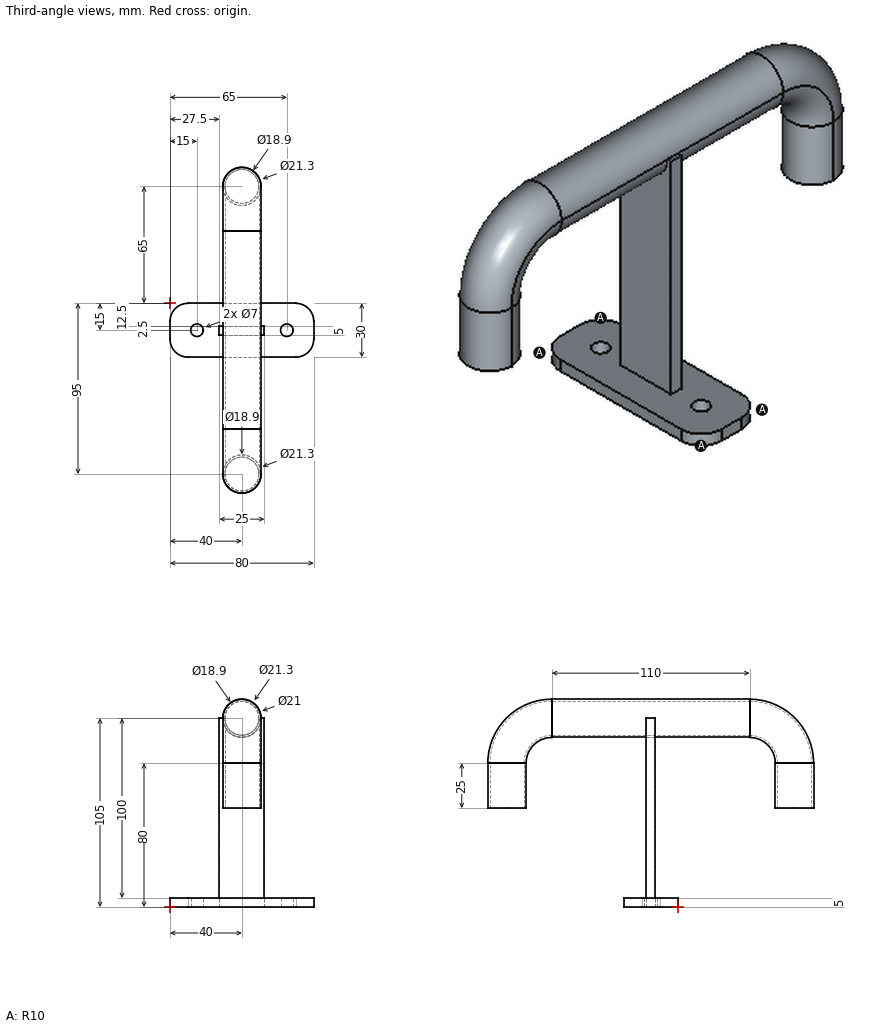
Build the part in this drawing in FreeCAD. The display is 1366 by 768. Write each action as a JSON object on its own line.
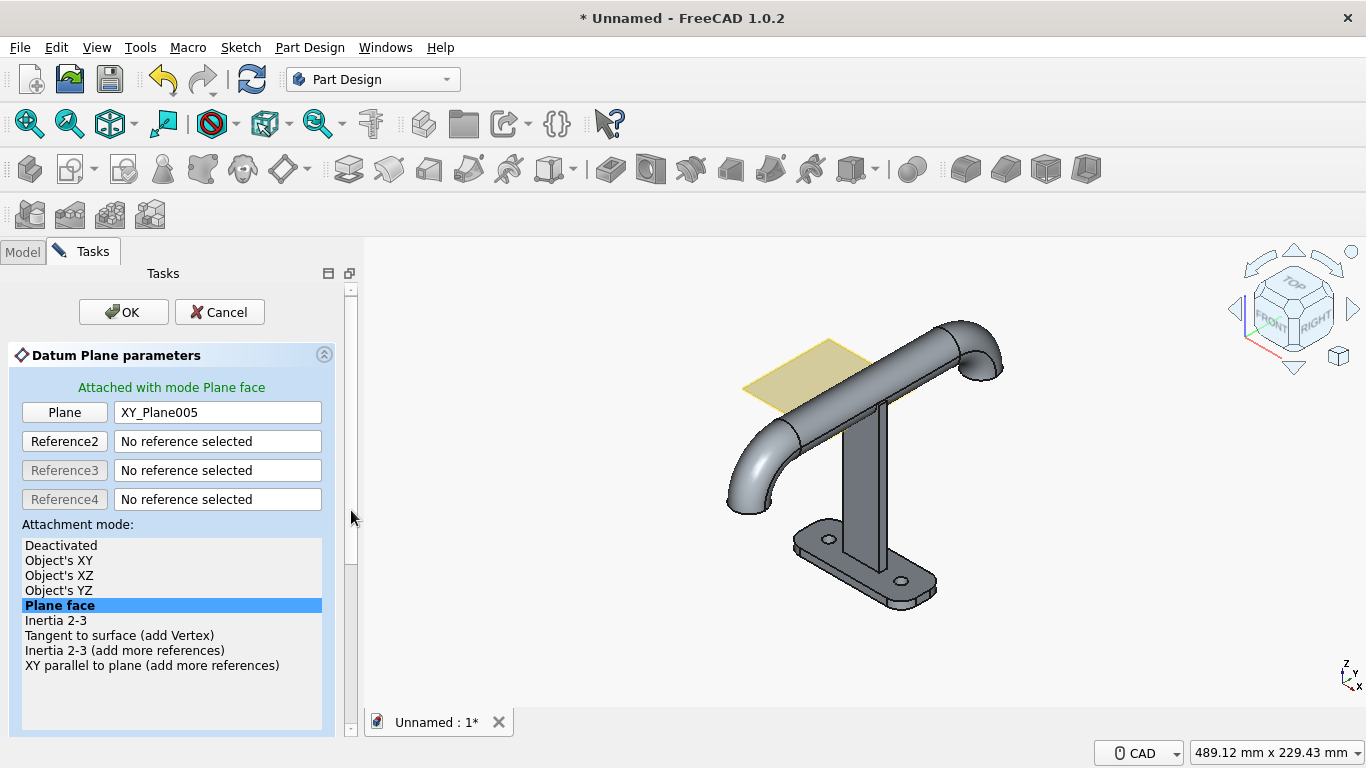
{"action": "left_click", "coordinate": [124, 312]}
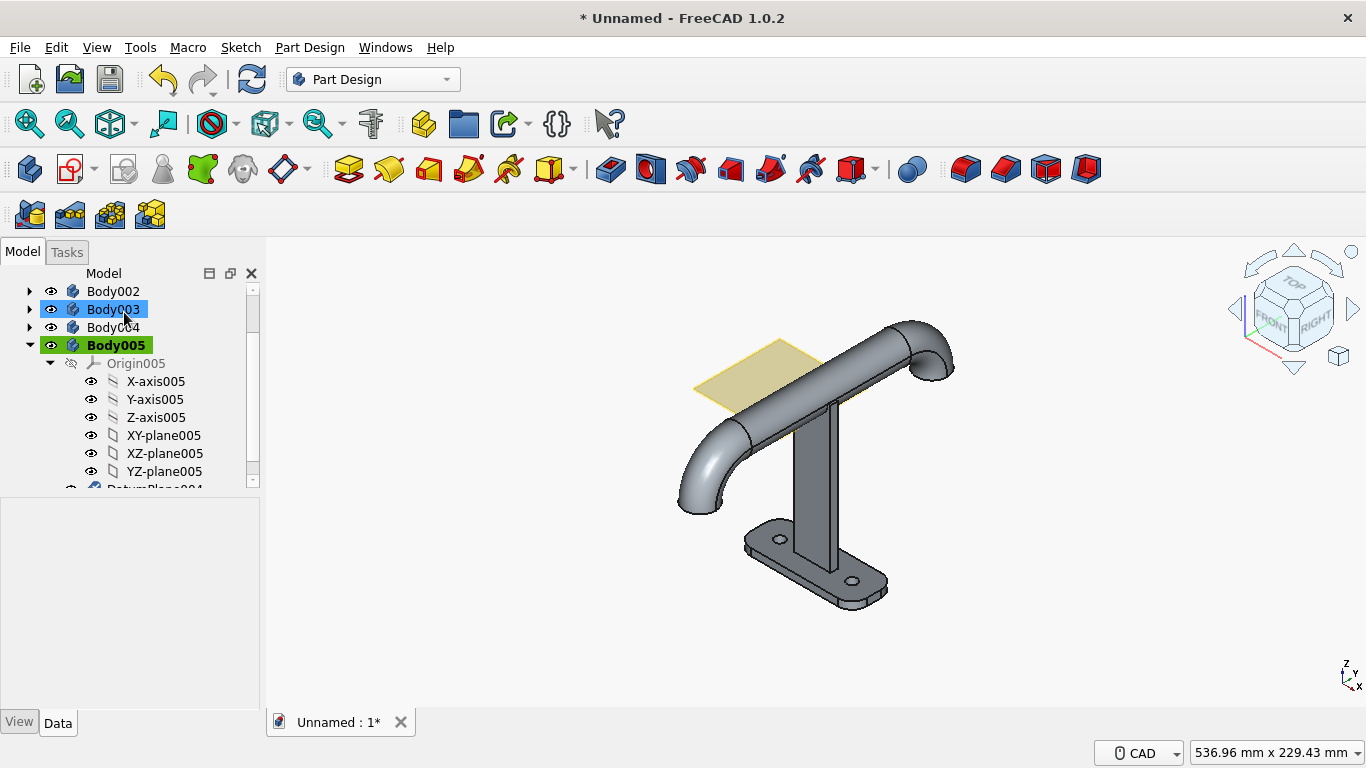
{"action": "scroll", "coordinate": [120, 377], "scroll_direction": "down", "scroll_amount": 3}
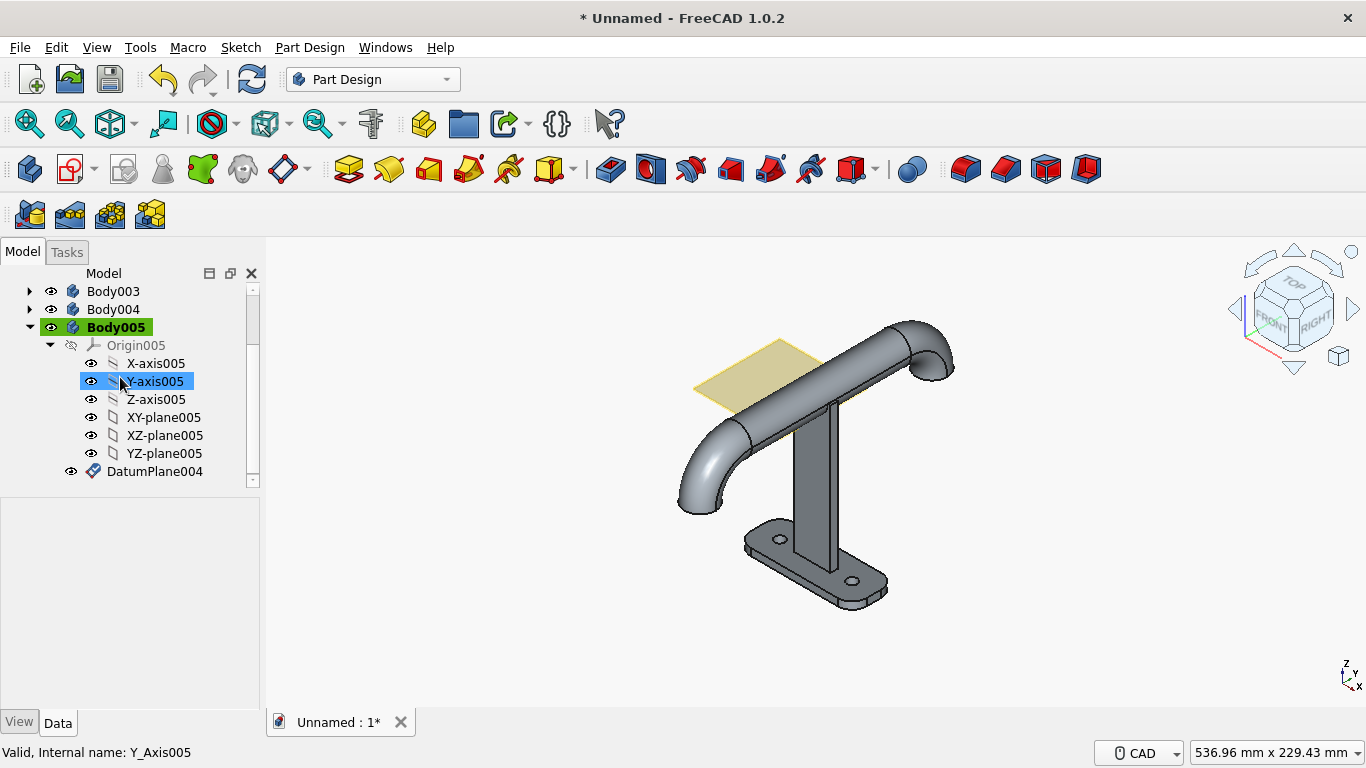
{"action": "left_click", "coordinate": [116, 471]}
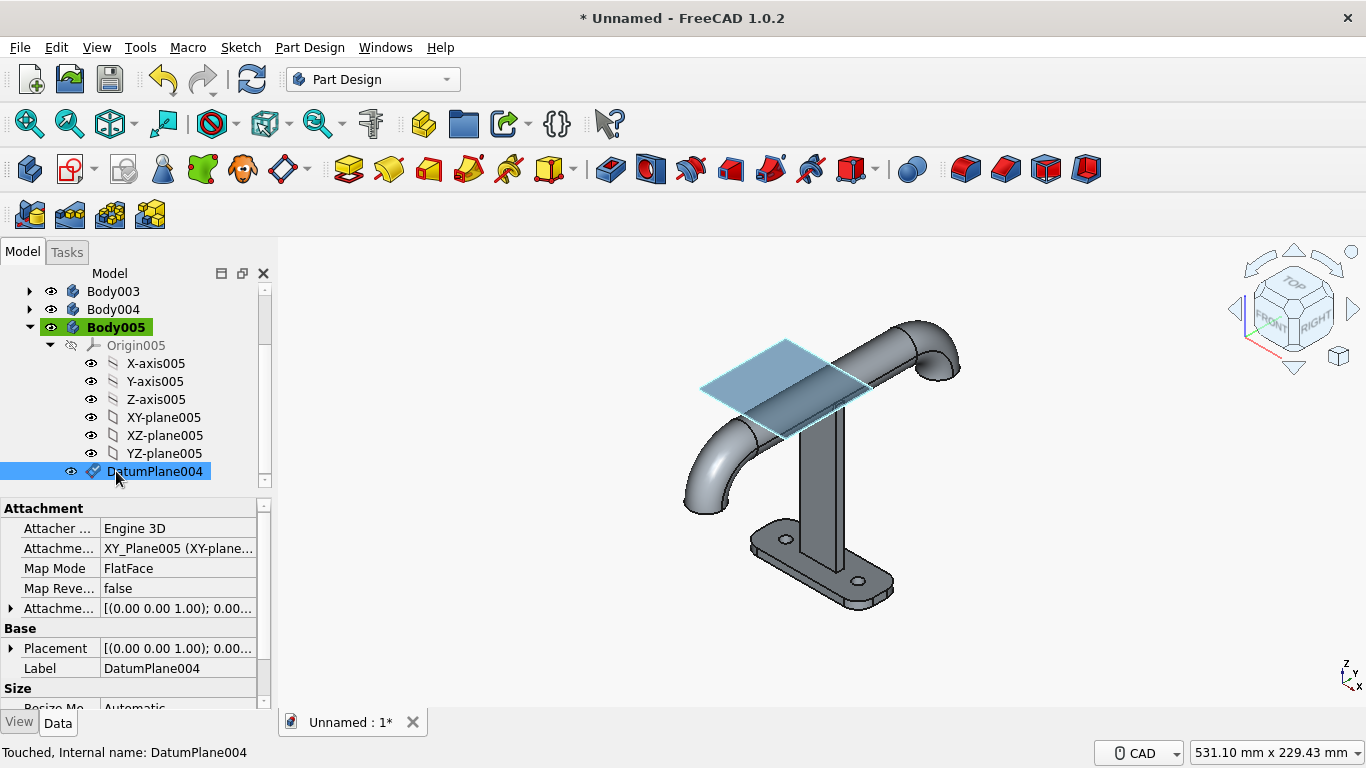
{"action": "left_click", "coordinate": [70, 170]}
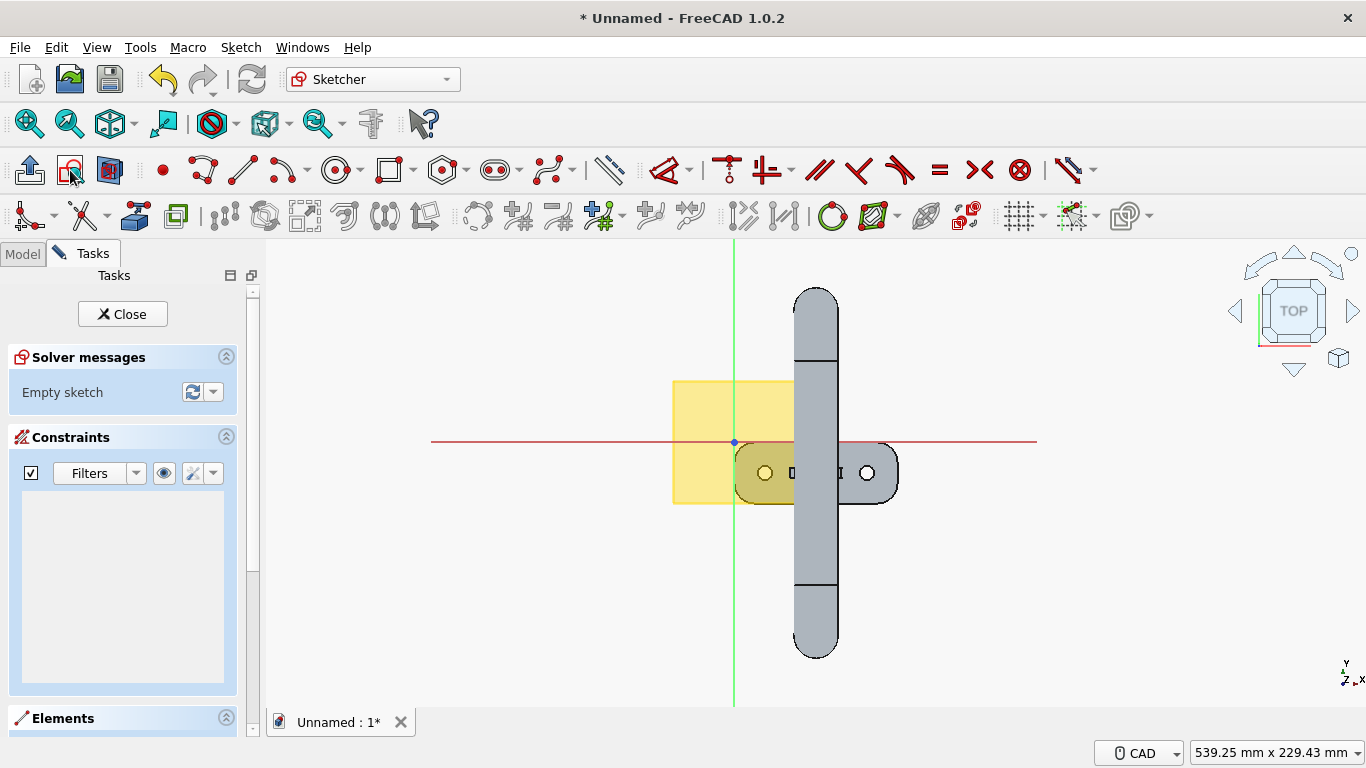
{"action": "scroll", "coordinate": [827, 662], "scroll_direction": "up", "scroll_amount": 10}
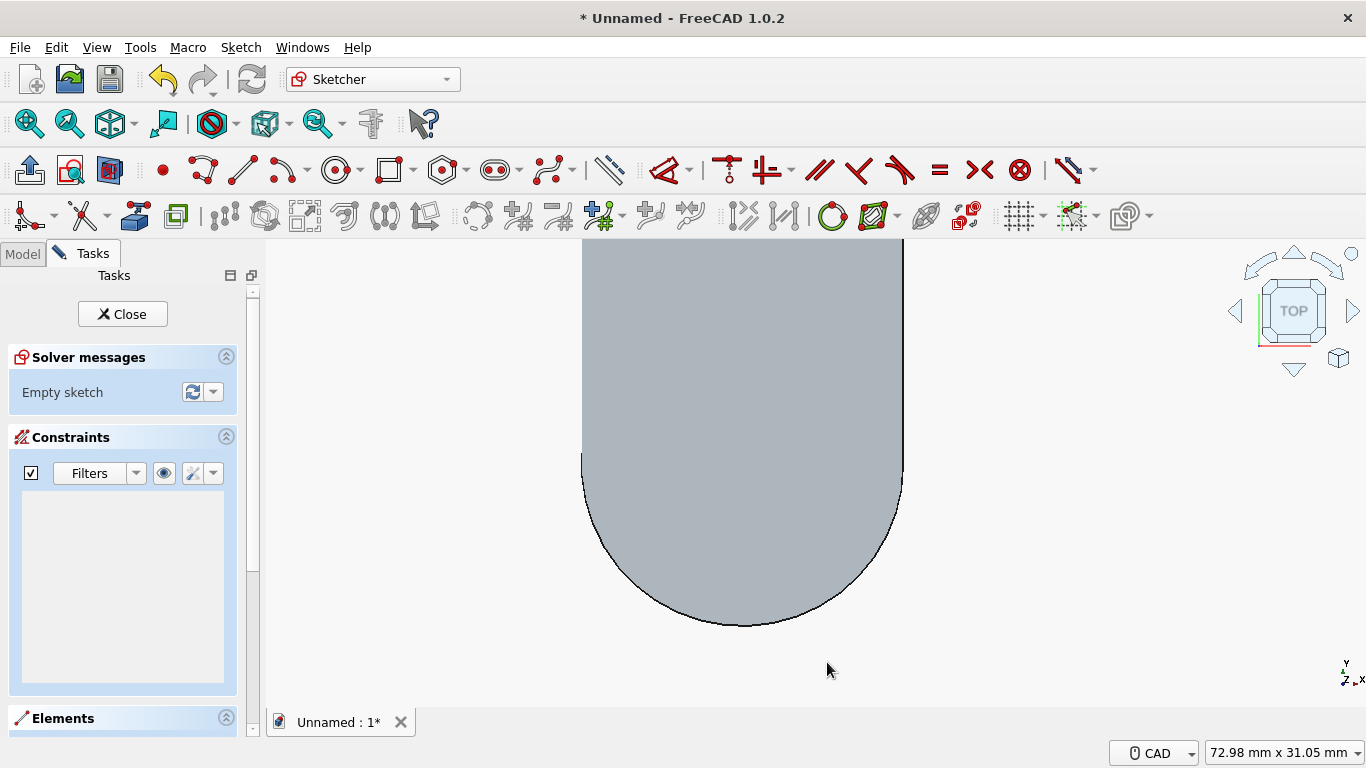
{"action": "left_click", "coordinate": [336, 170]}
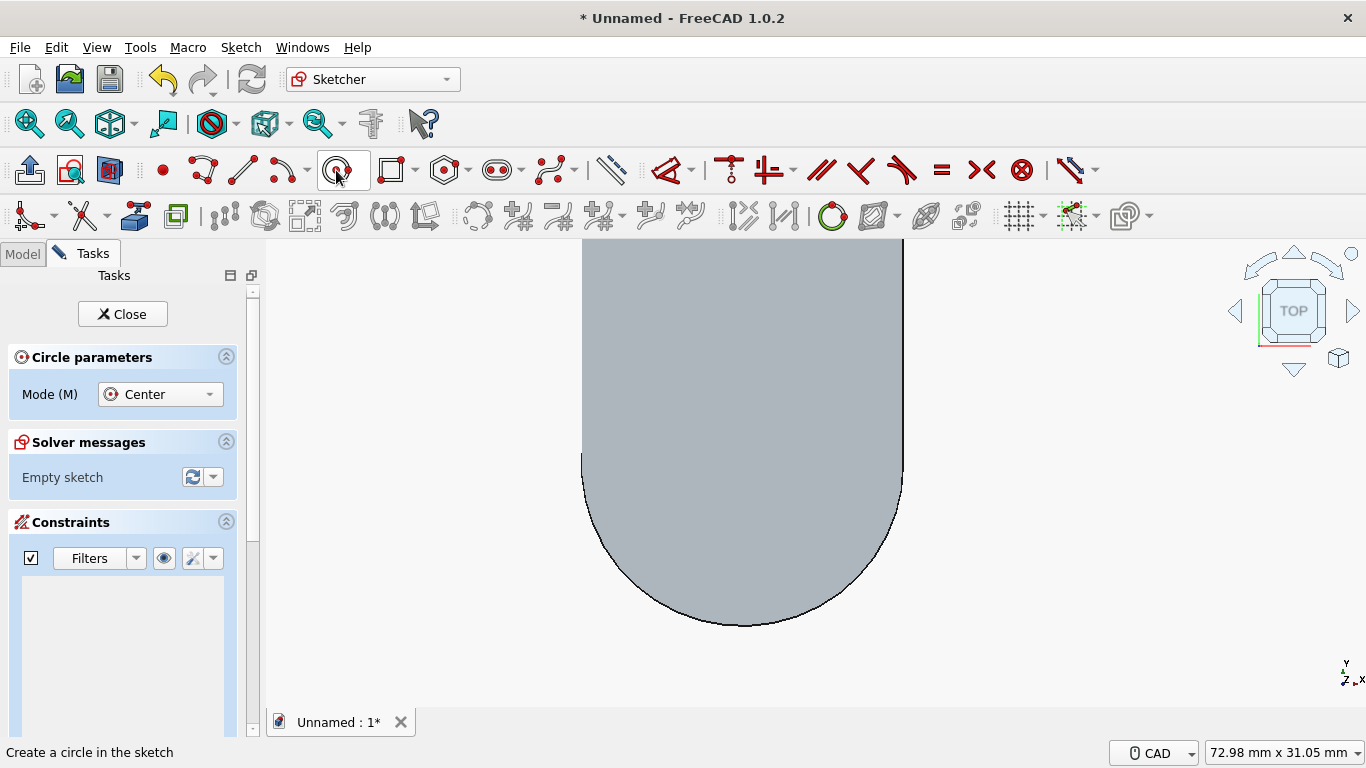
{"action": "left_click", "coordinate": [742, 465]}
{"action": "mouse_move", "coordinate": [856, 352]}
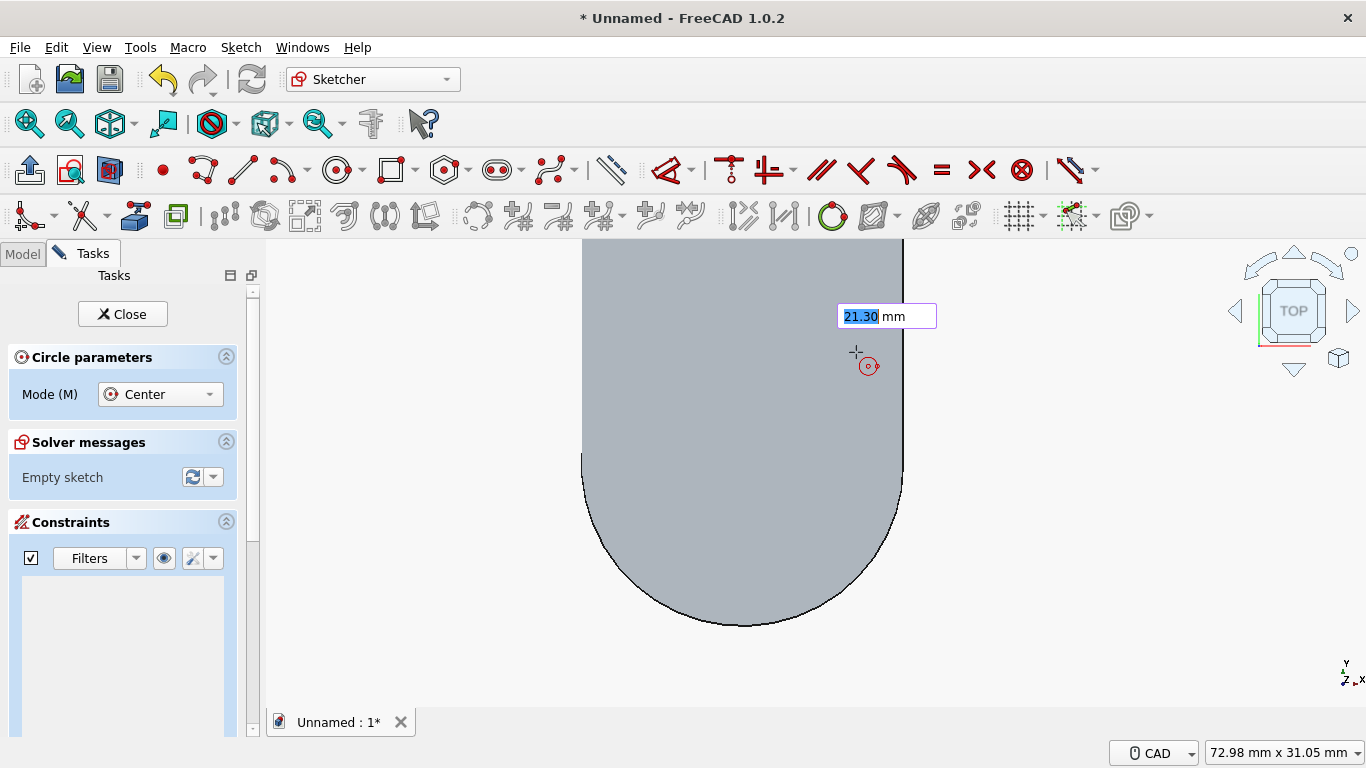
{"action": "type", "text": "21.3"}
{"action": "key", "text": "Return"}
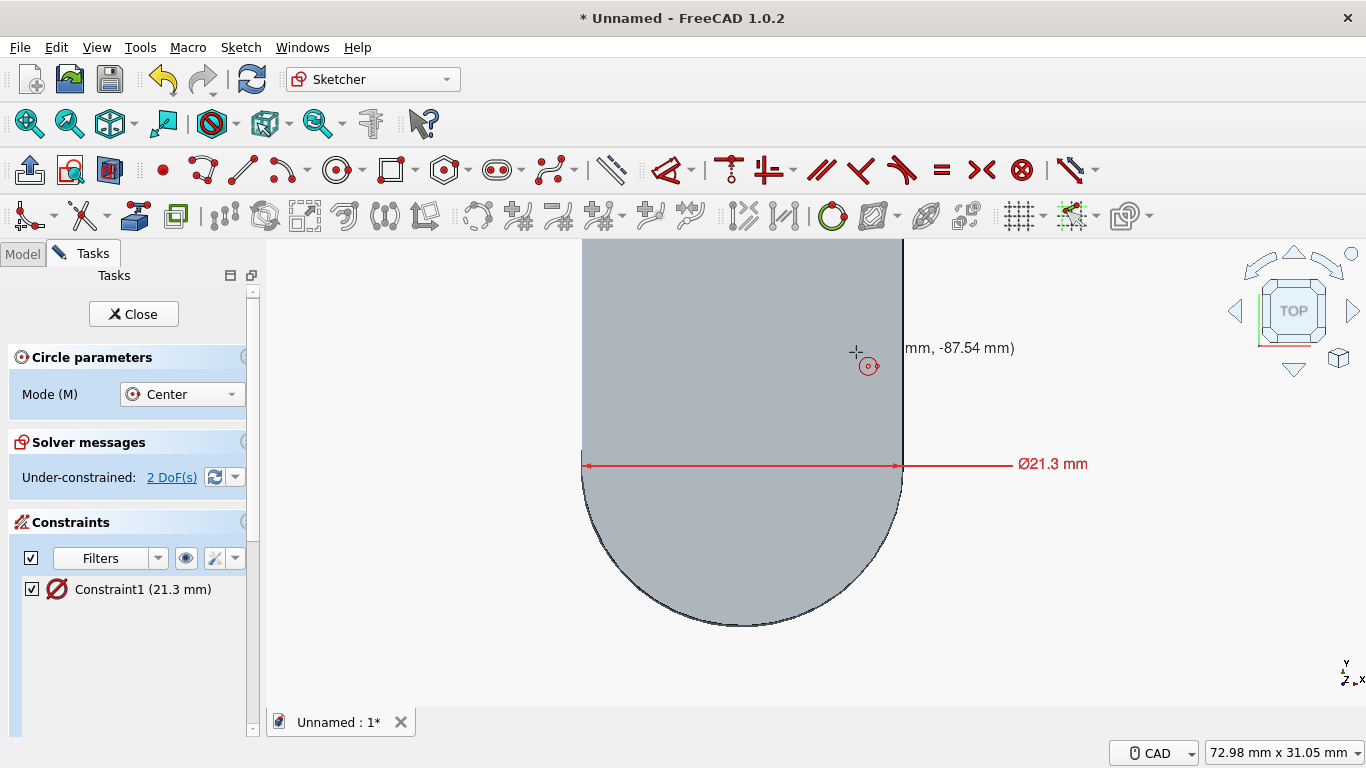
{"action": "left_click", "coordinate": [742, 466]}
{"action": "mouse_move", "coordinate": [843, 365]}